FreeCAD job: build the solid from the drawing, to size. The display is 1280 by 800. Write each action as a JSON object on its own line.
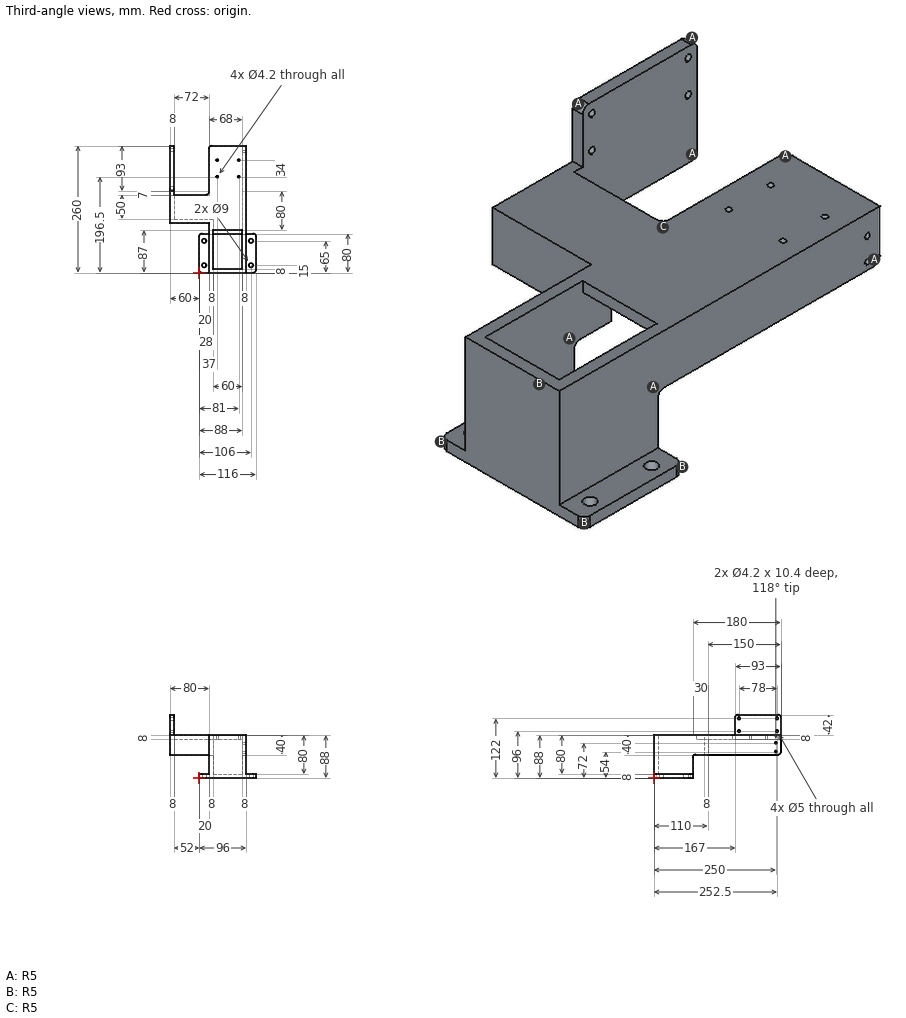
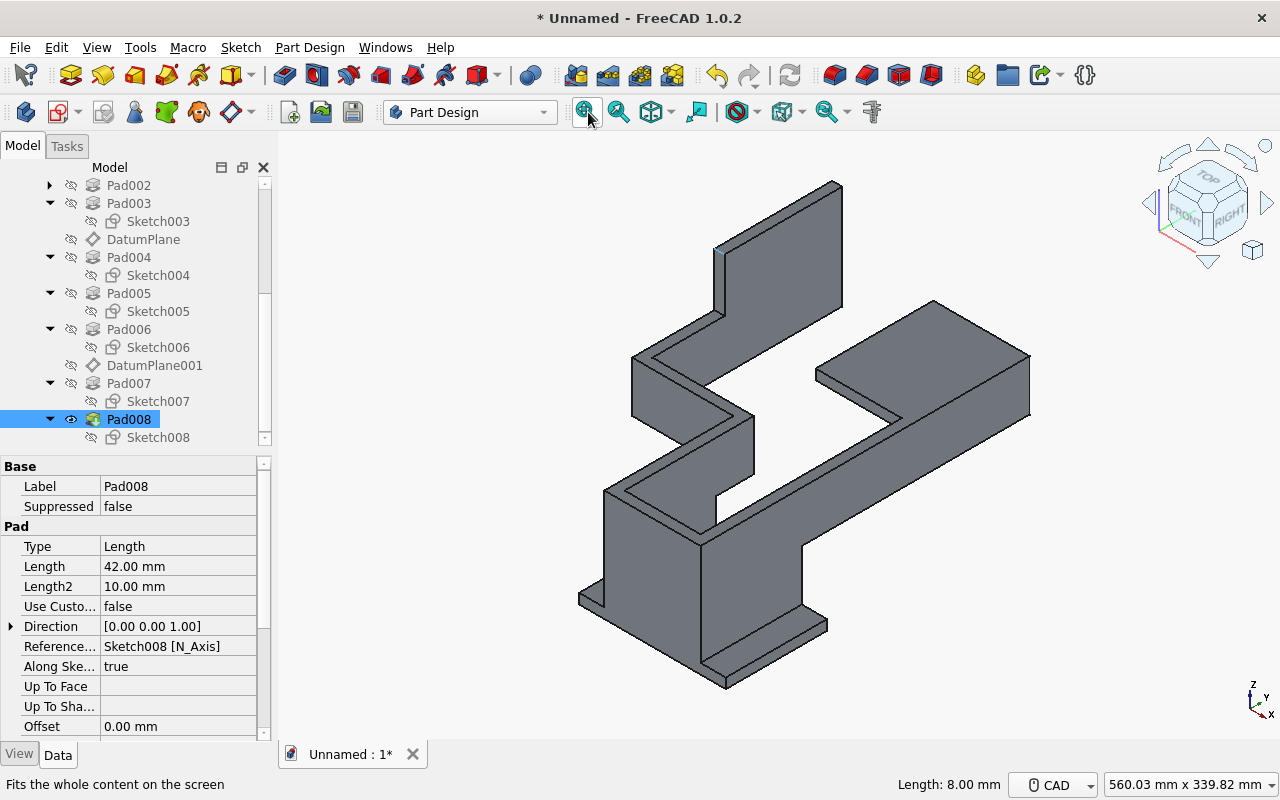
{"action": "key", "text": "2"}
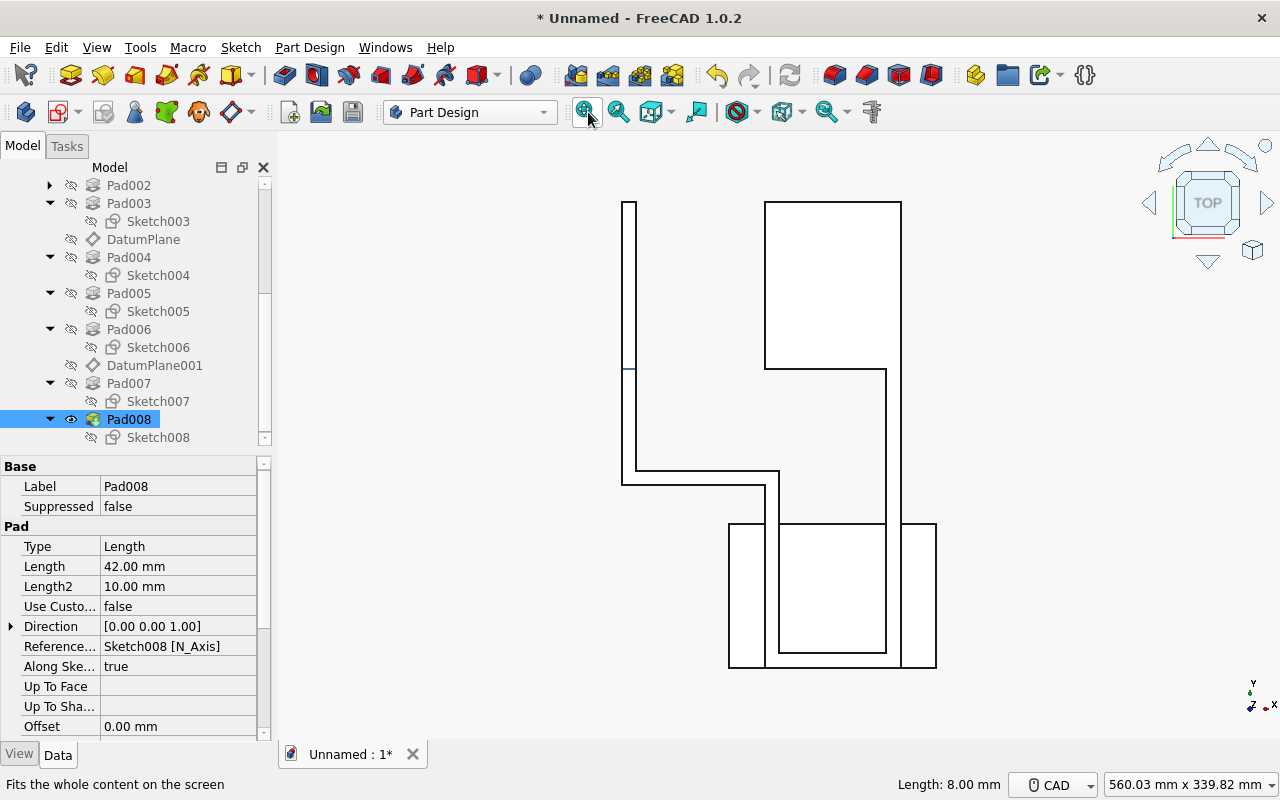
{"action": "left_click", "coordinate": [629, 201], "text": "ctrl"}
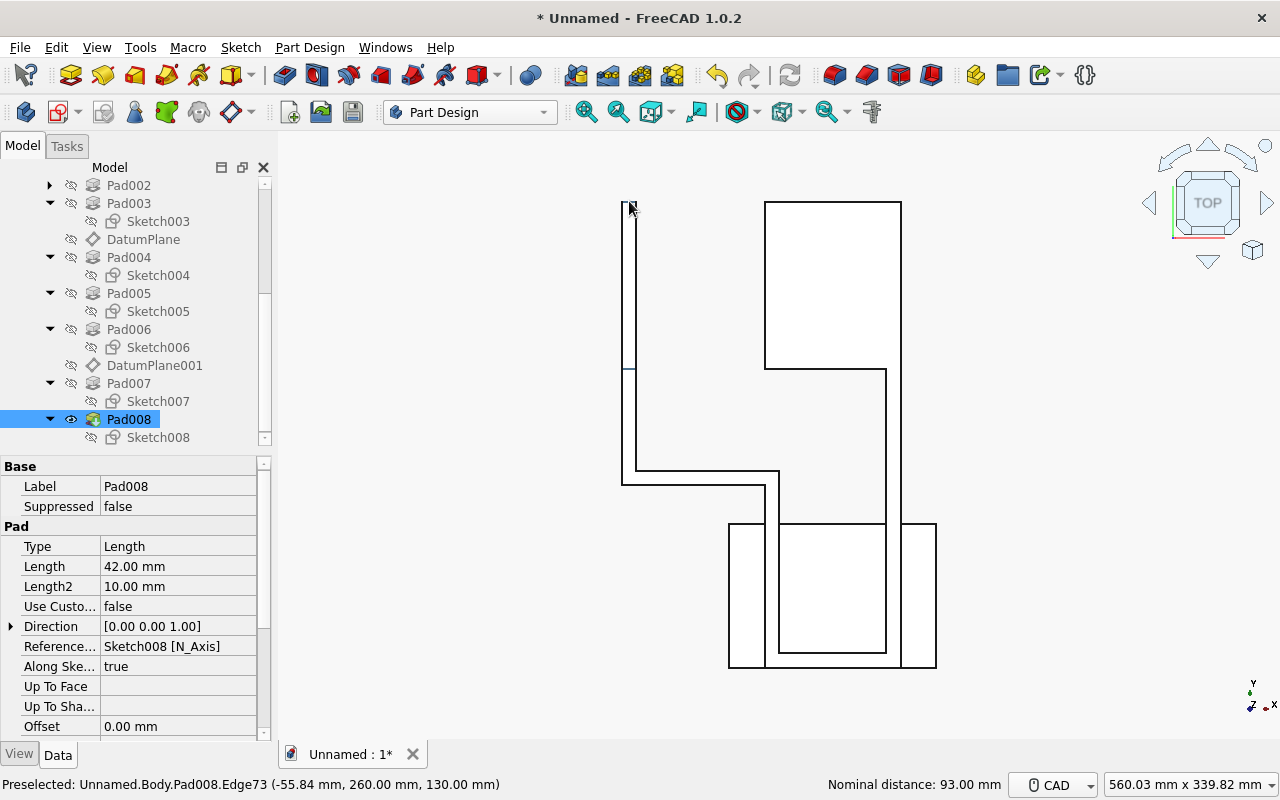
{"action": "scroll", "coordinate": [629, 201], "scroll_direction": "up", "scroll_amount": 6}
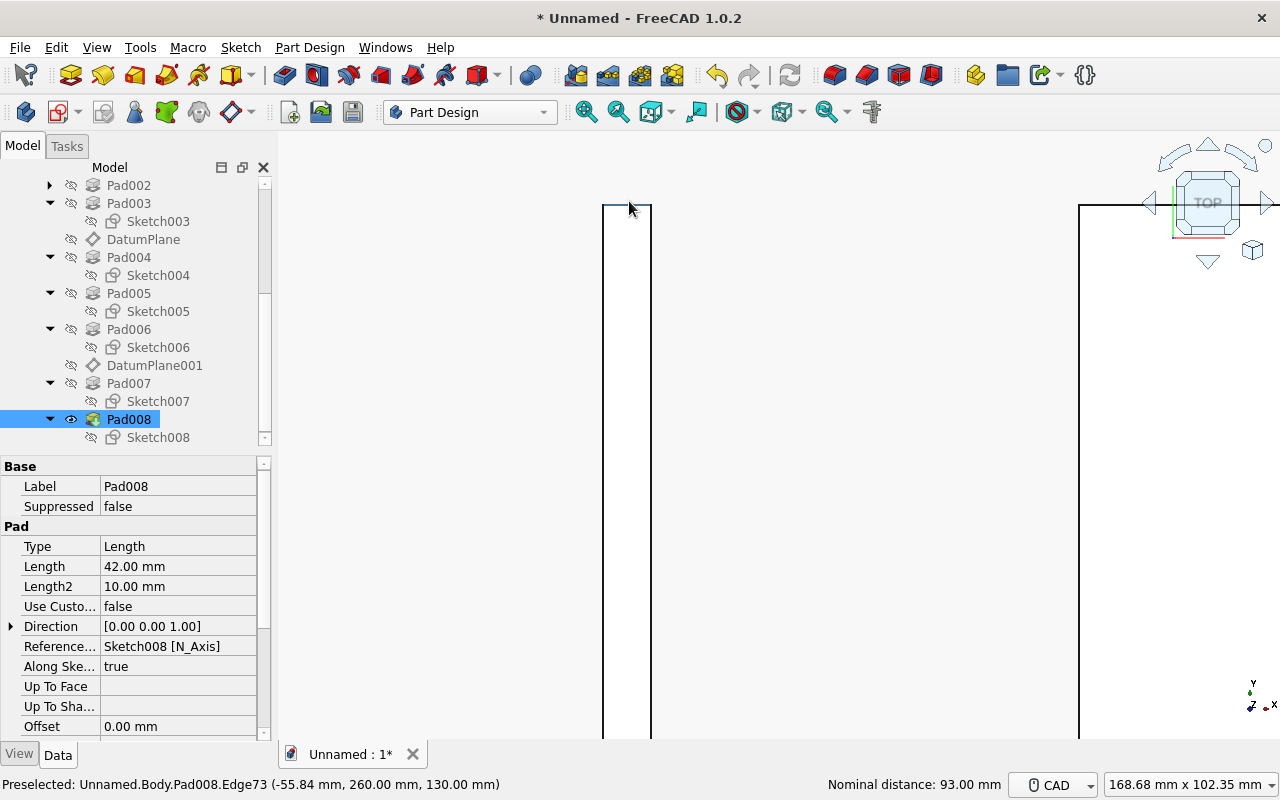
{"action": "left_click", "coordinate": [588, 112]}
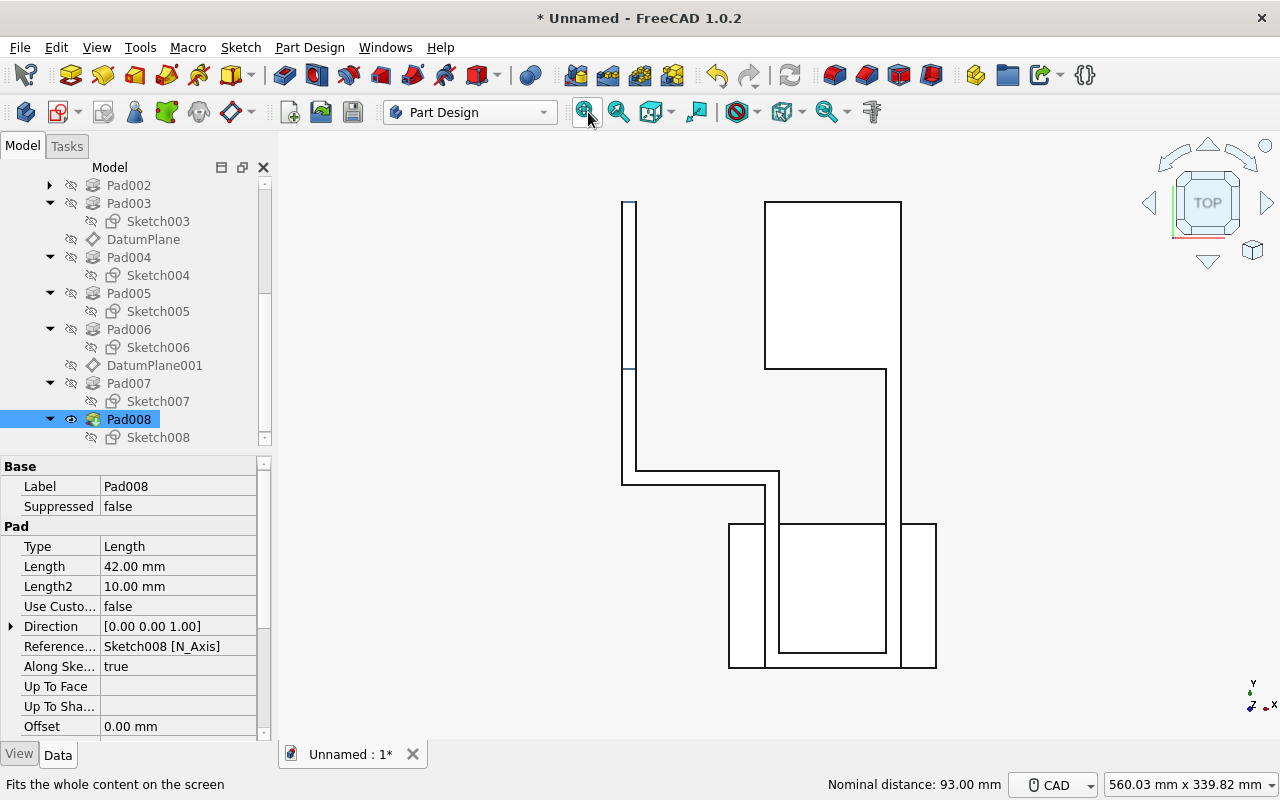
{"action": "key", "text": "0"}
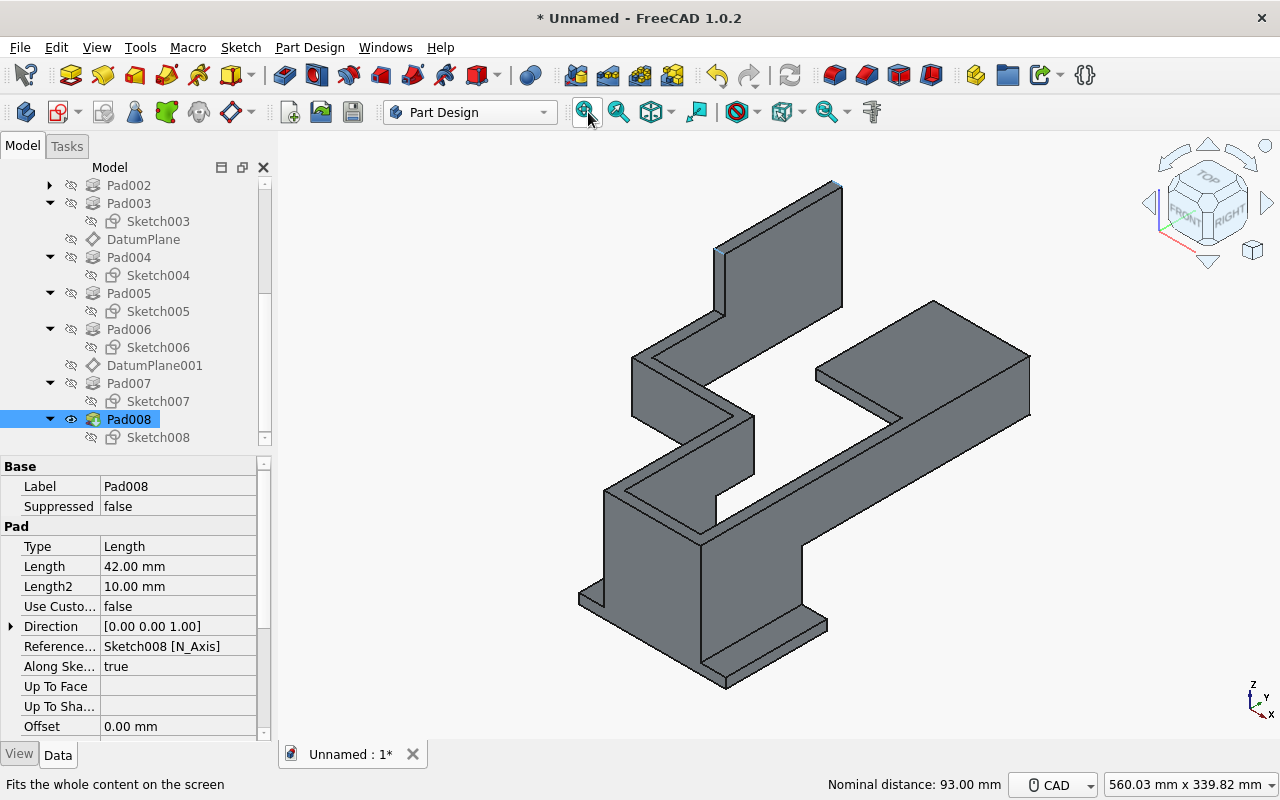
{"action": "scroll", "coordinate": [837, 303], "scroll_direction": "up", "scroll_amount": 6}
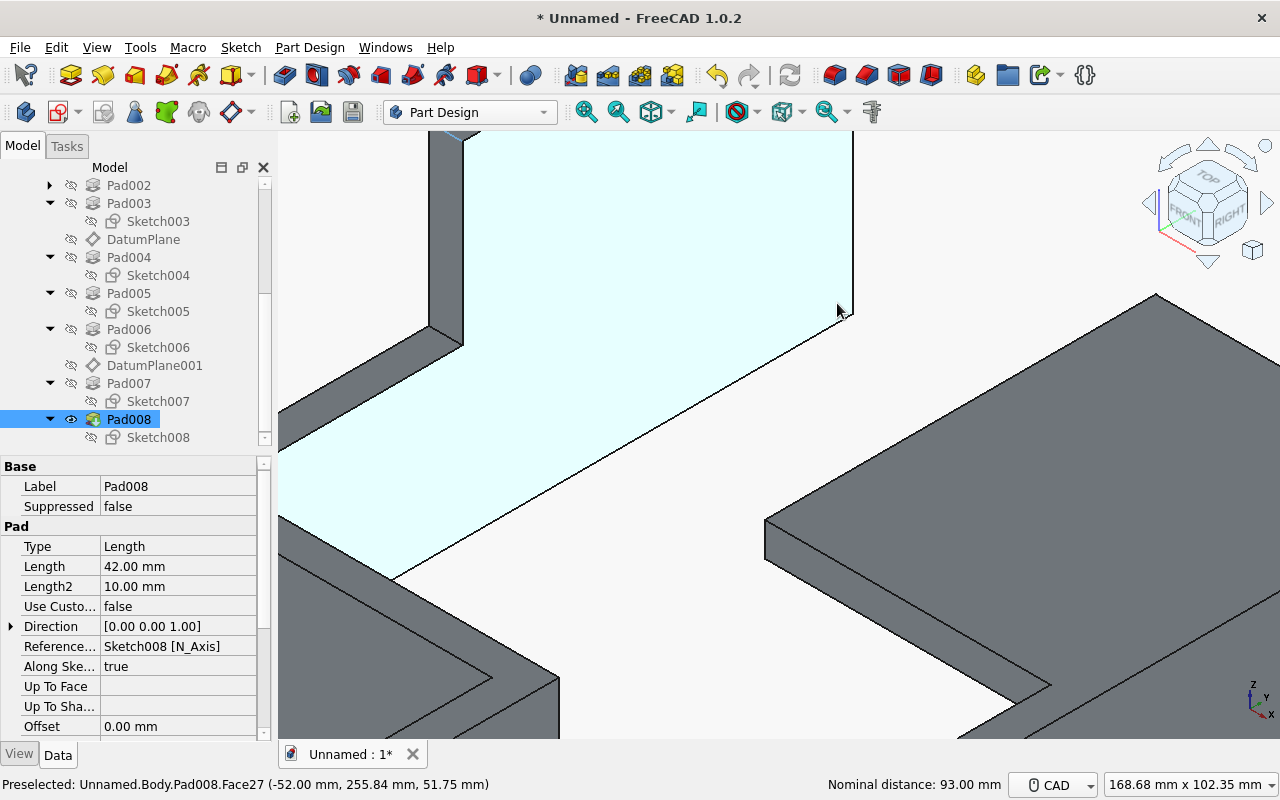
{"action": "left_click", "coordinate": [588, 112]}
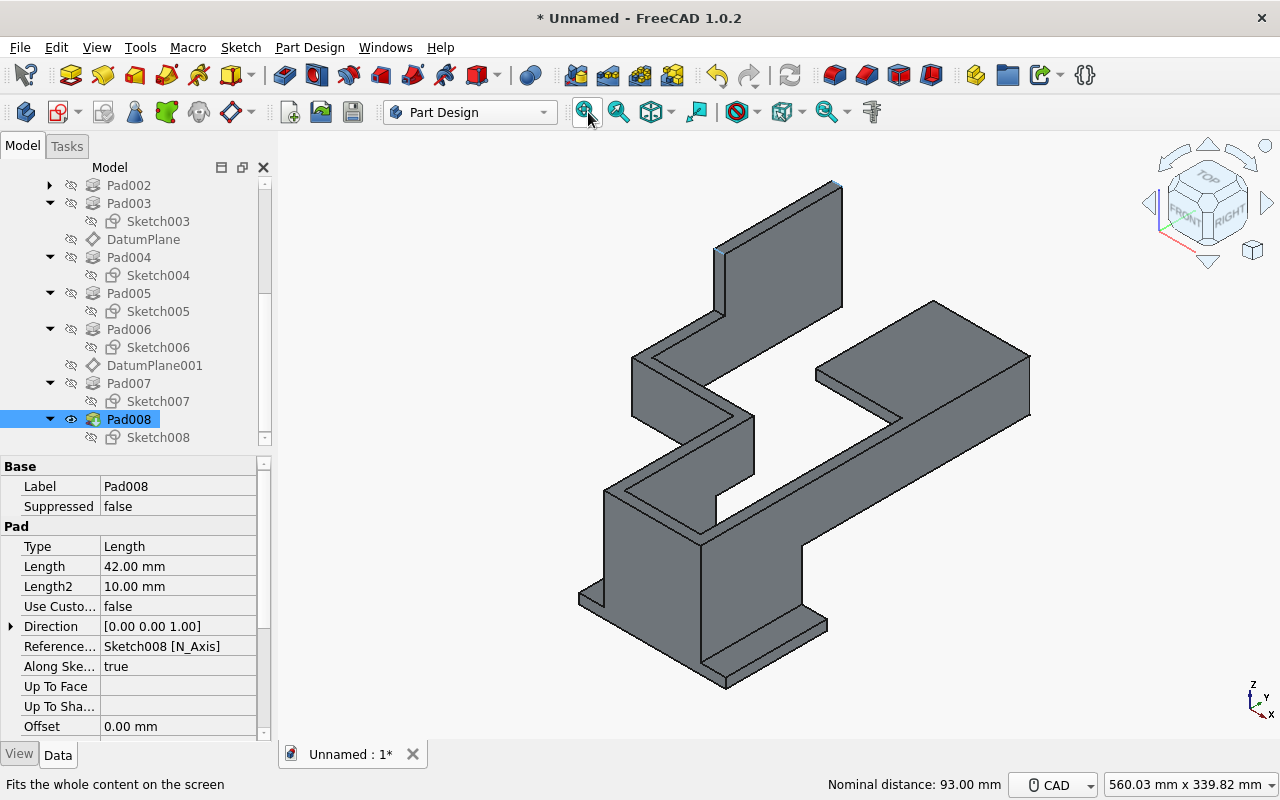
{"action": "key", "text": "1"}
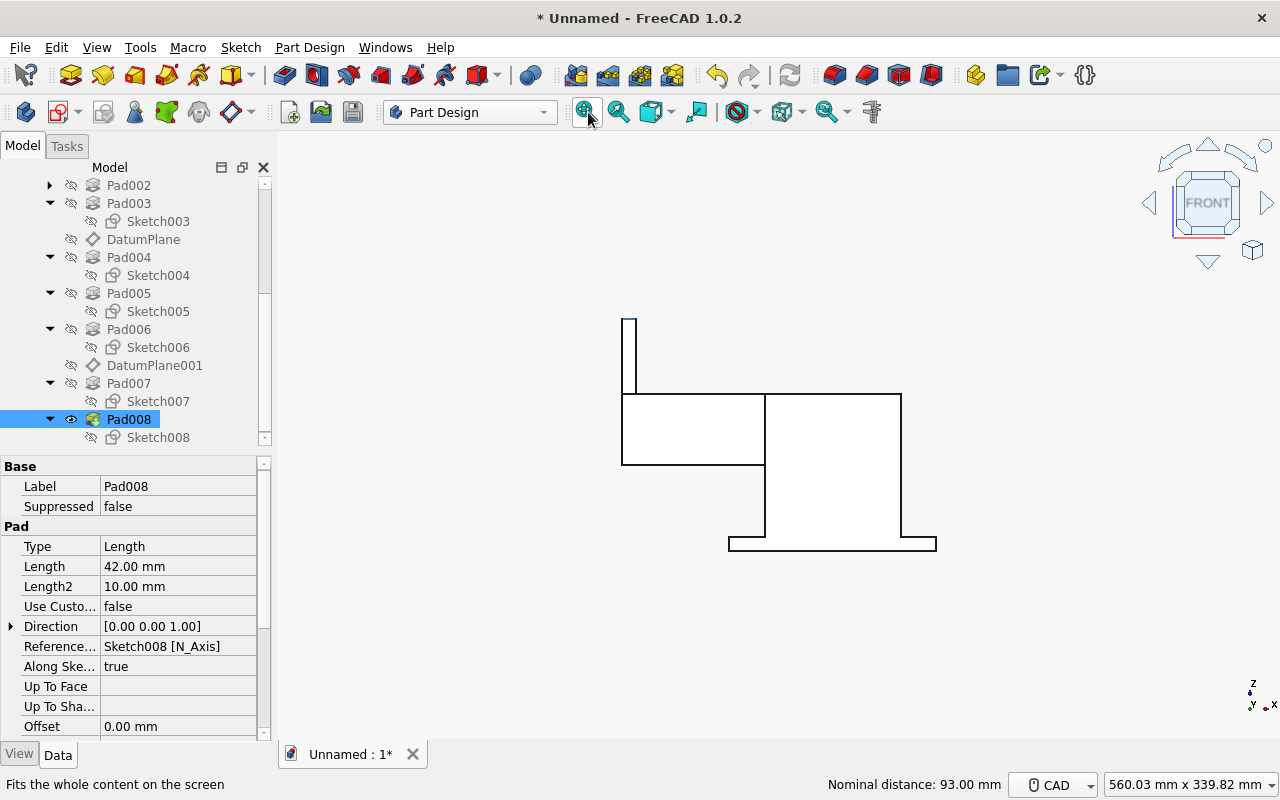
{"action": "left_click", "coordinate": [588, 112]}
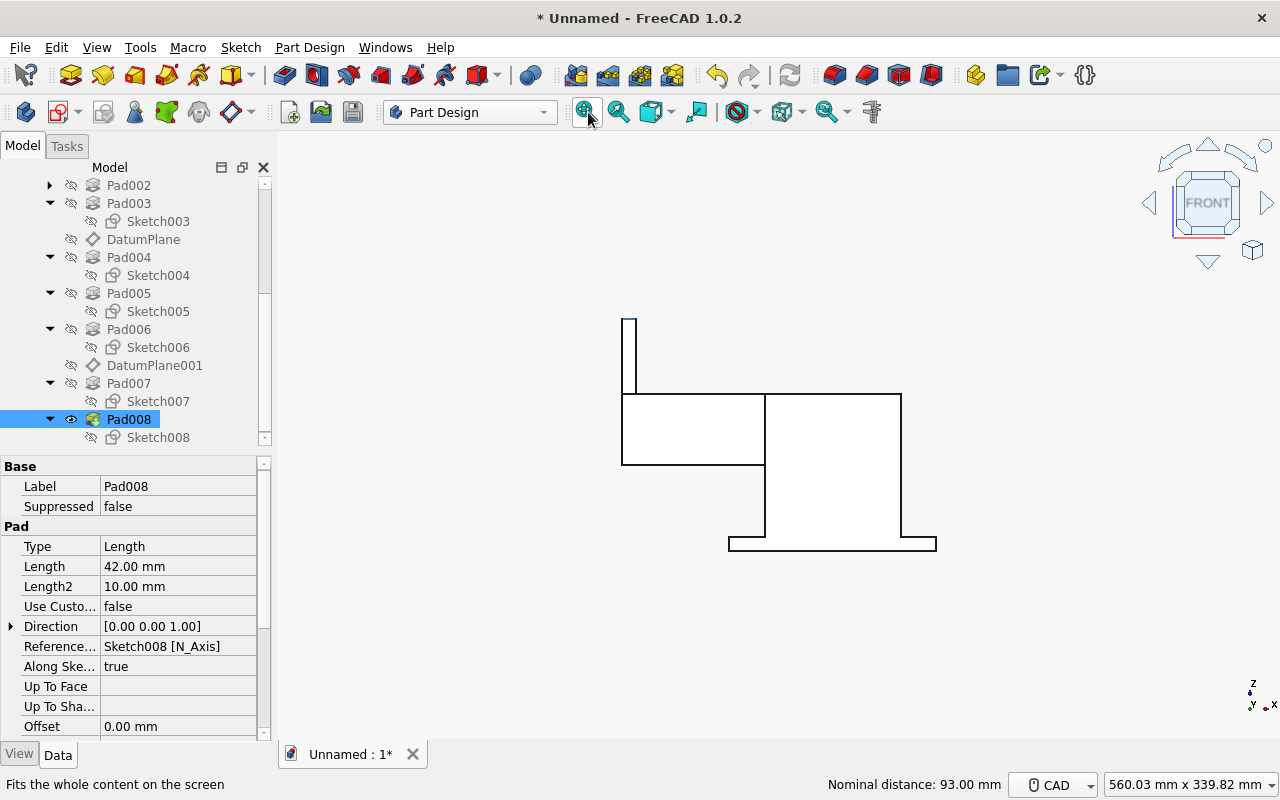
{"action": "scroll", "coordinate": [629, 464], "scroll_direction": "up", "scroll_amount": 6}